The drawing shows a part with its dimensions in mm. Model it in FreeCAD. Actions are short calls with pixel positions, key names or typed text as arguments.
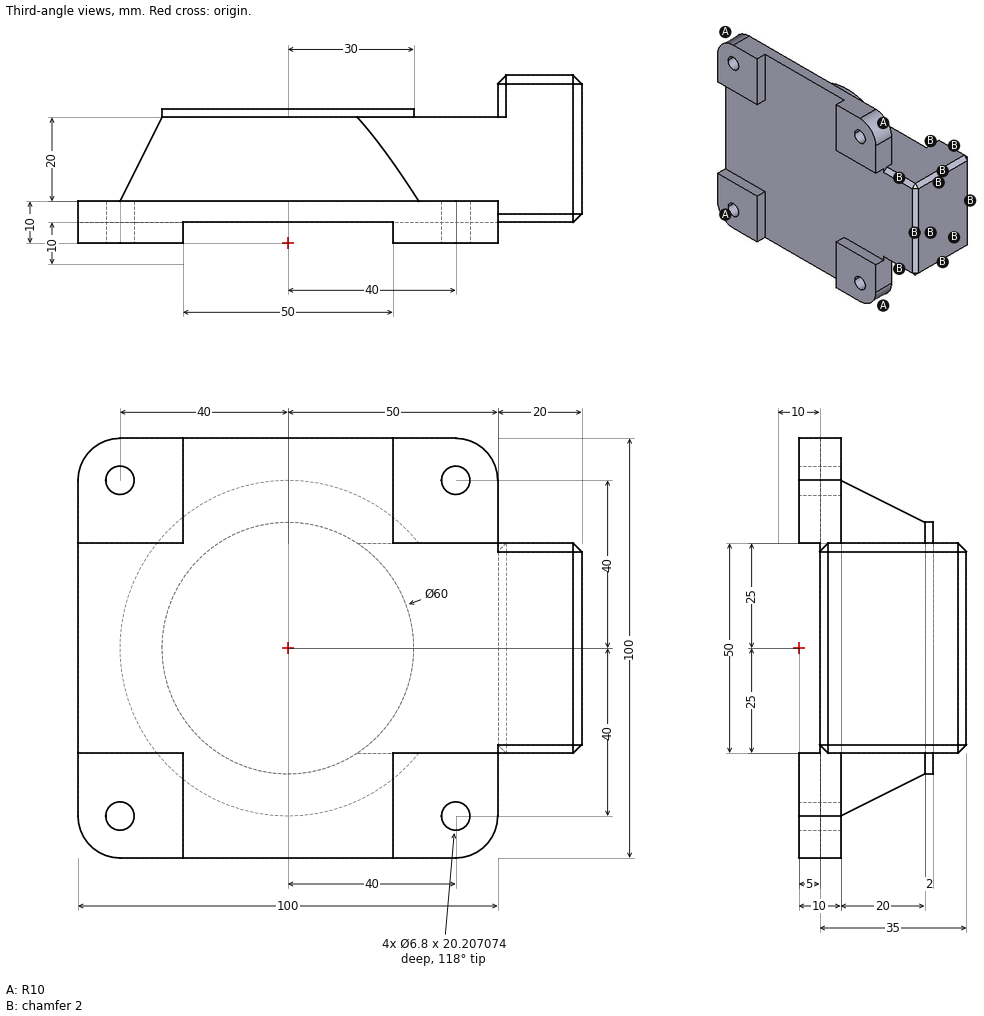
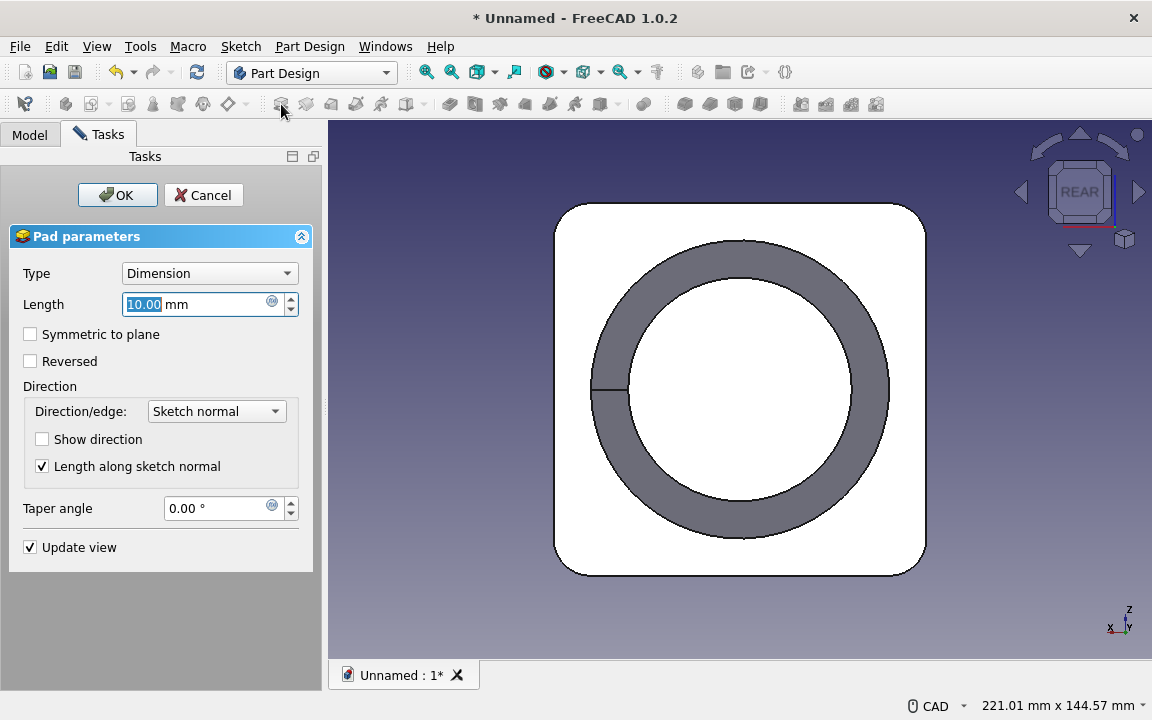
text(2)
key(Tab)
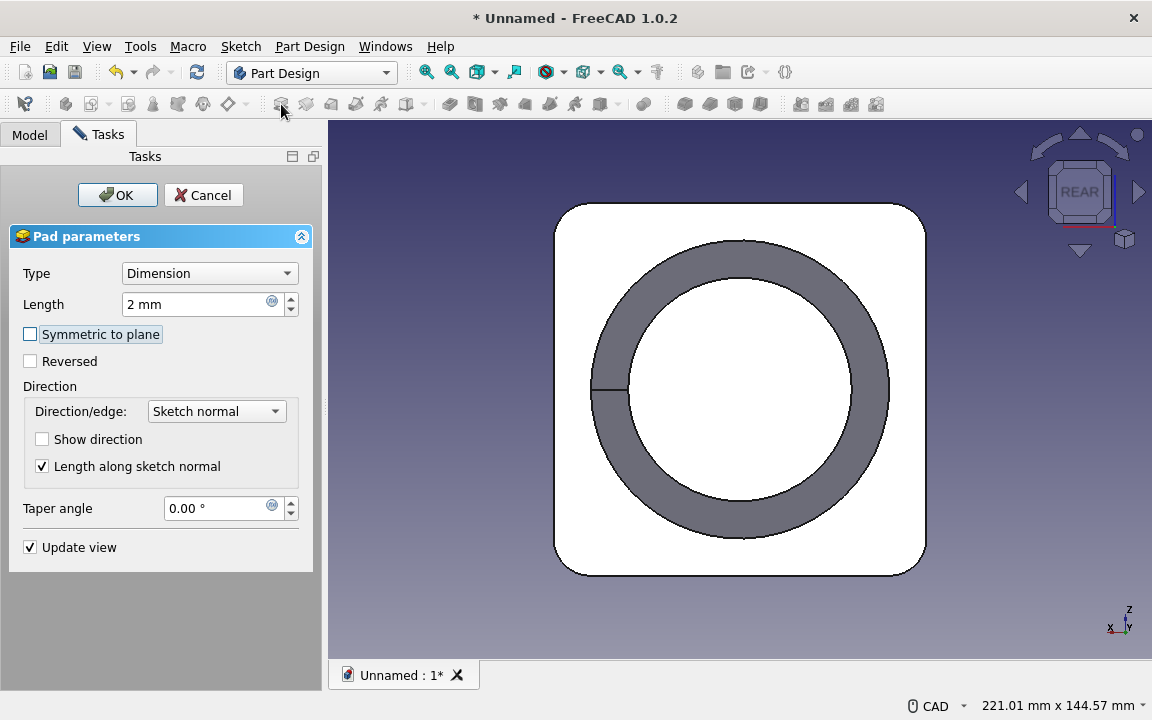
click(118, 195)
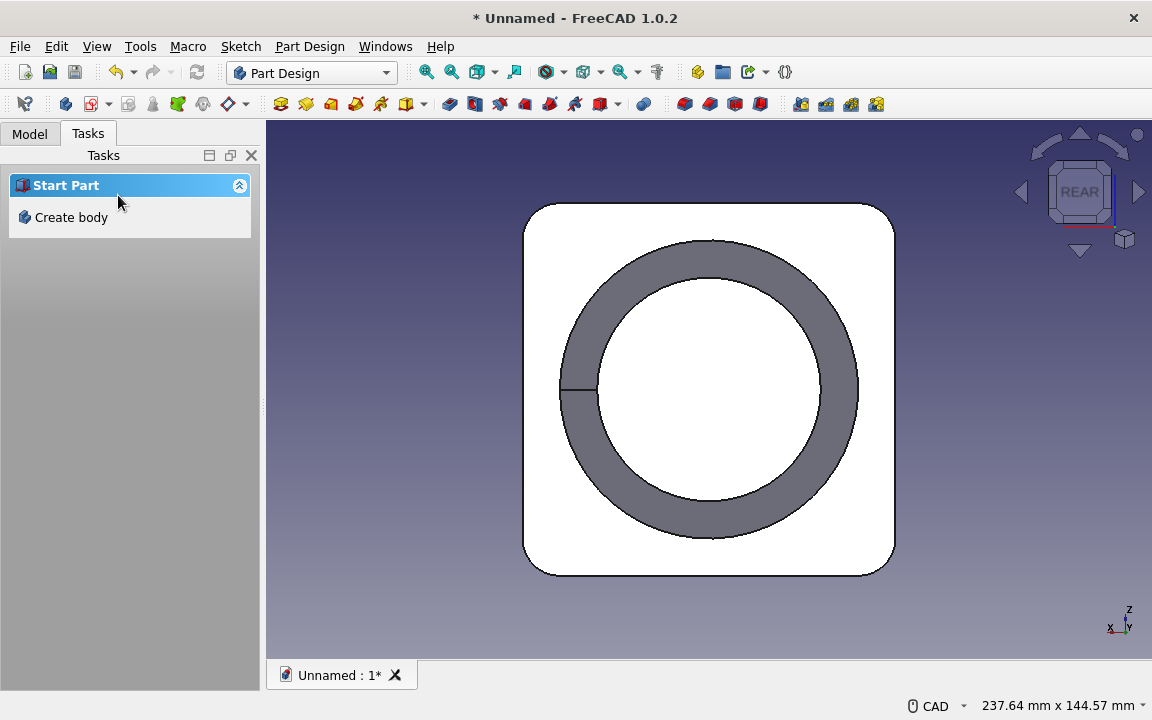
click(90, 104)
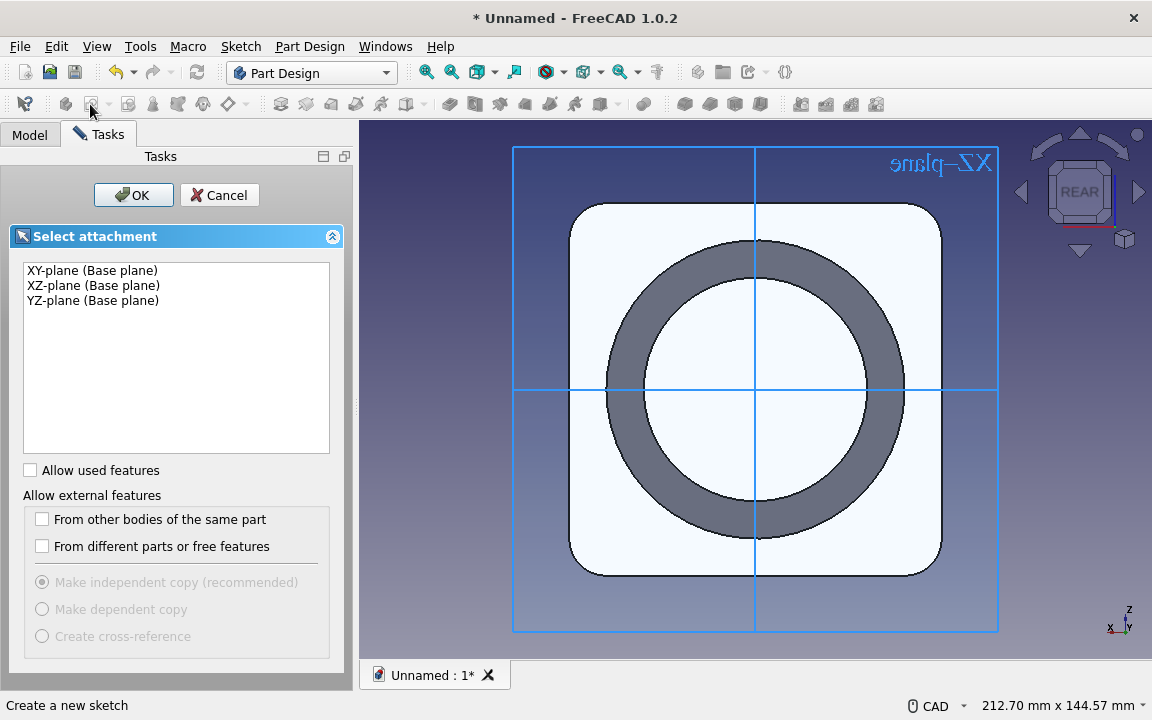
click(84, 300)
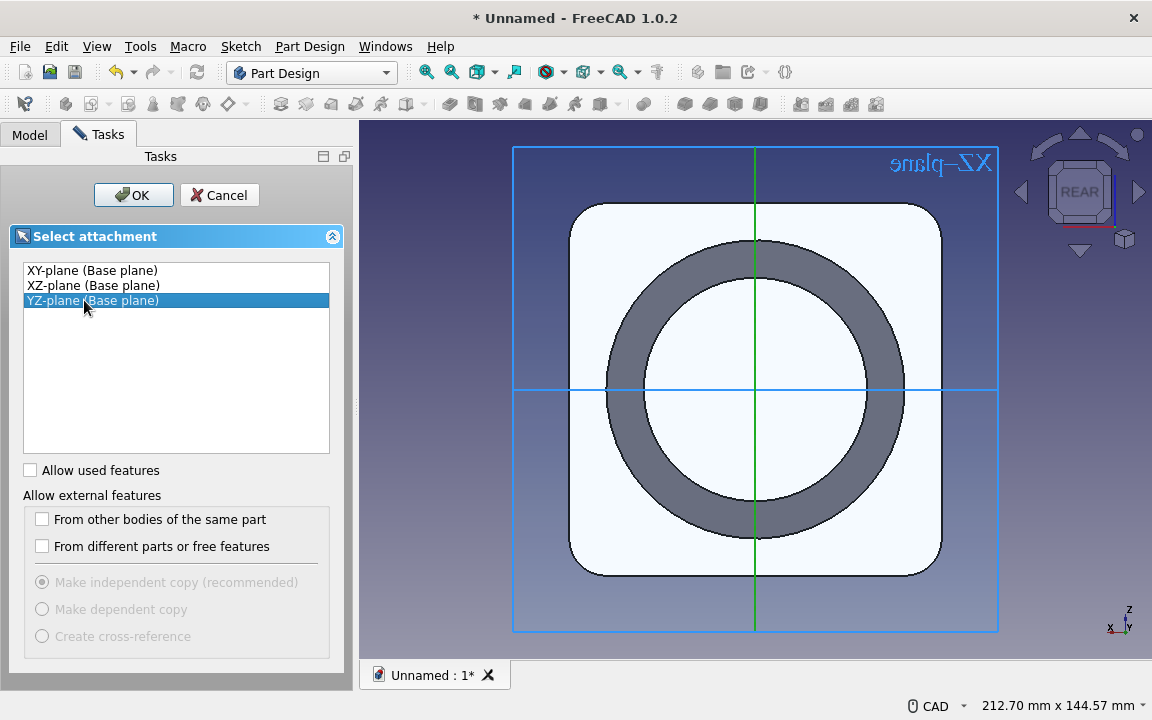
click(134, 195)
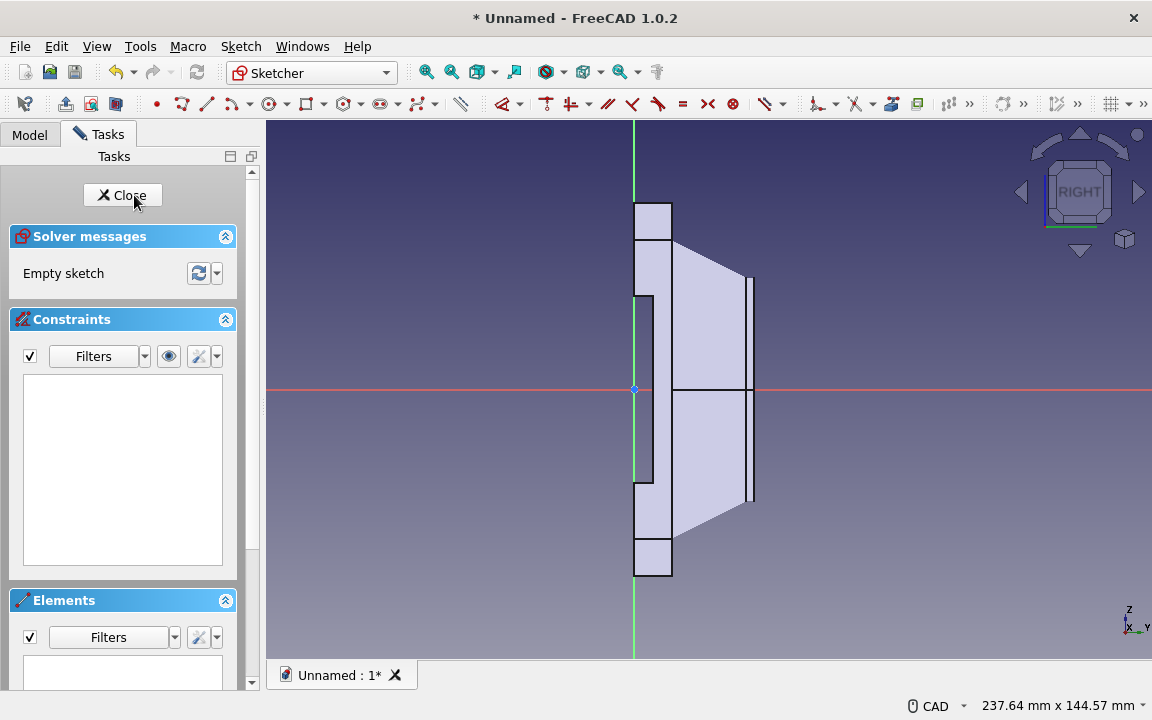
key(q)
key(s)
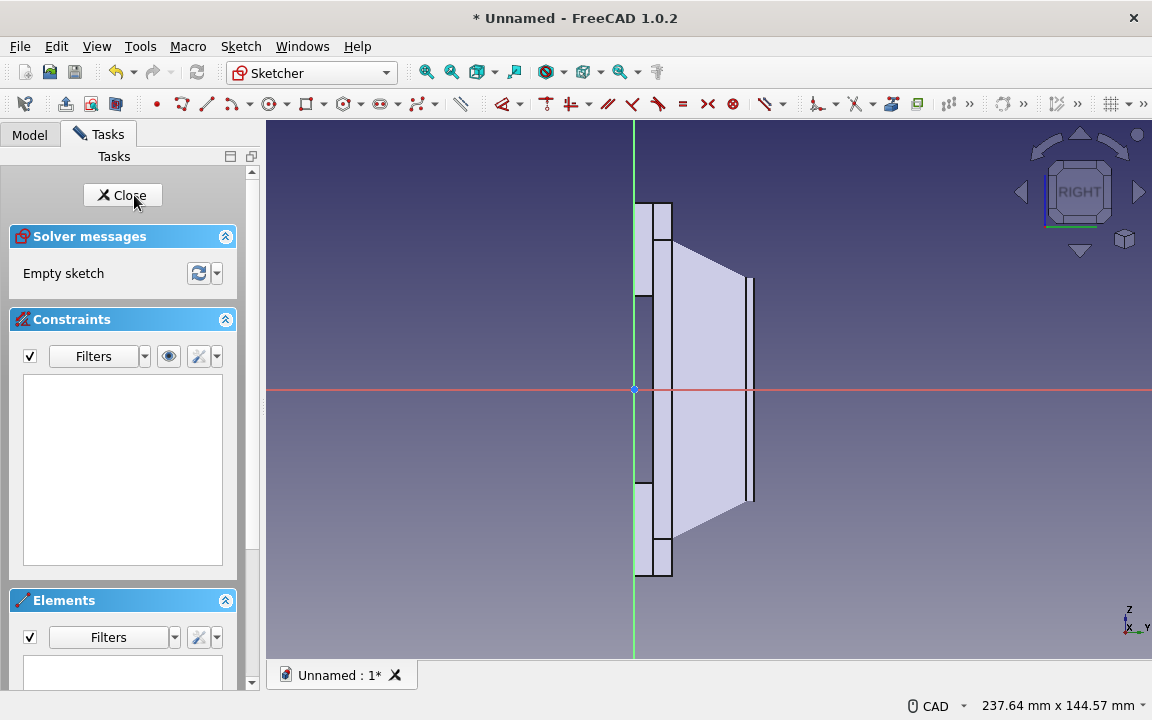
scroll(751, 390, up, 3)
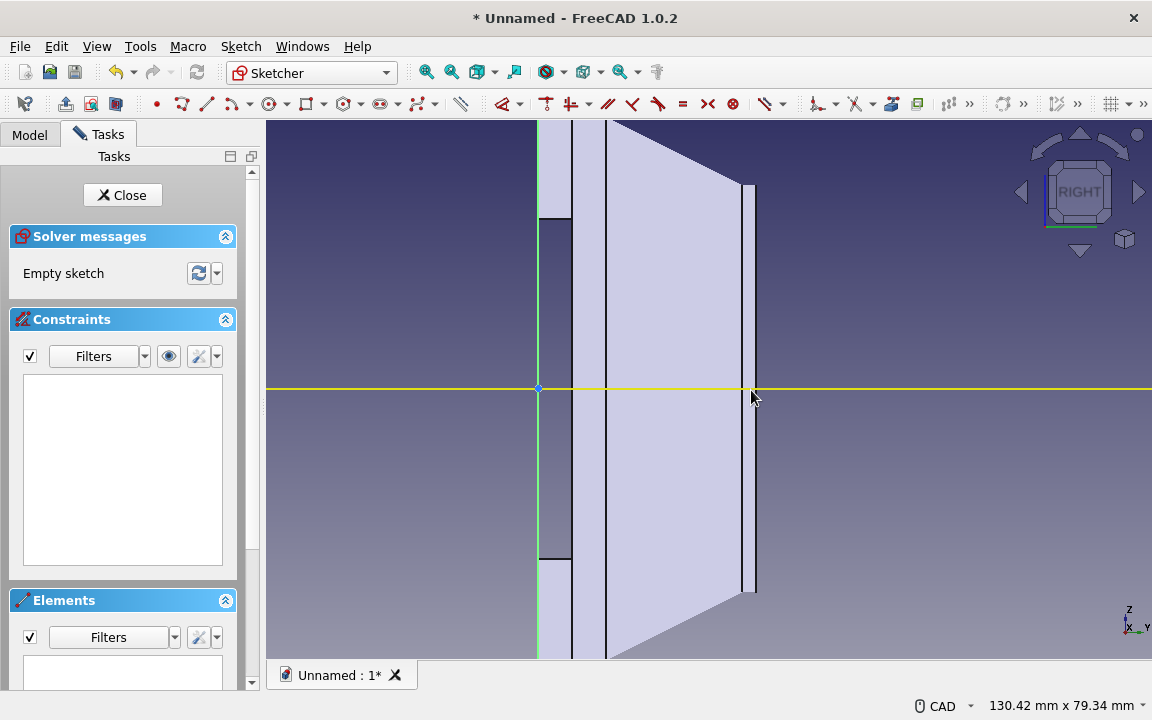
click(306, 104)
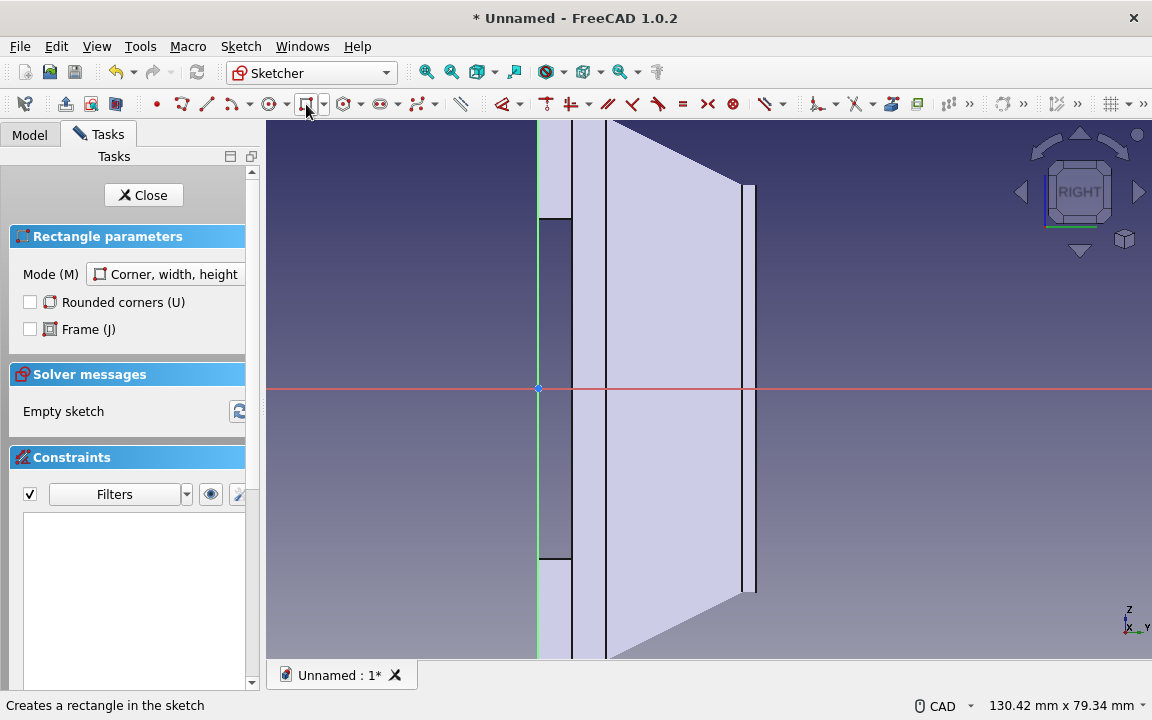
click(606, 219)
click(742, 559)
key(Escape)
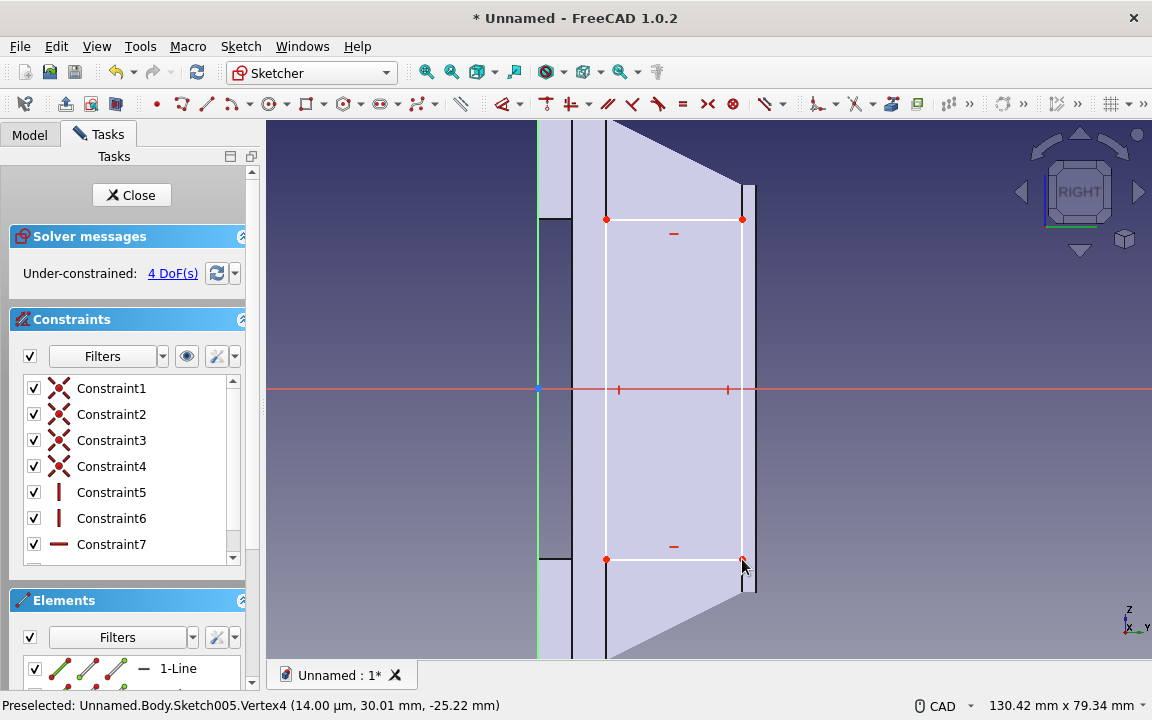
click(502, 104)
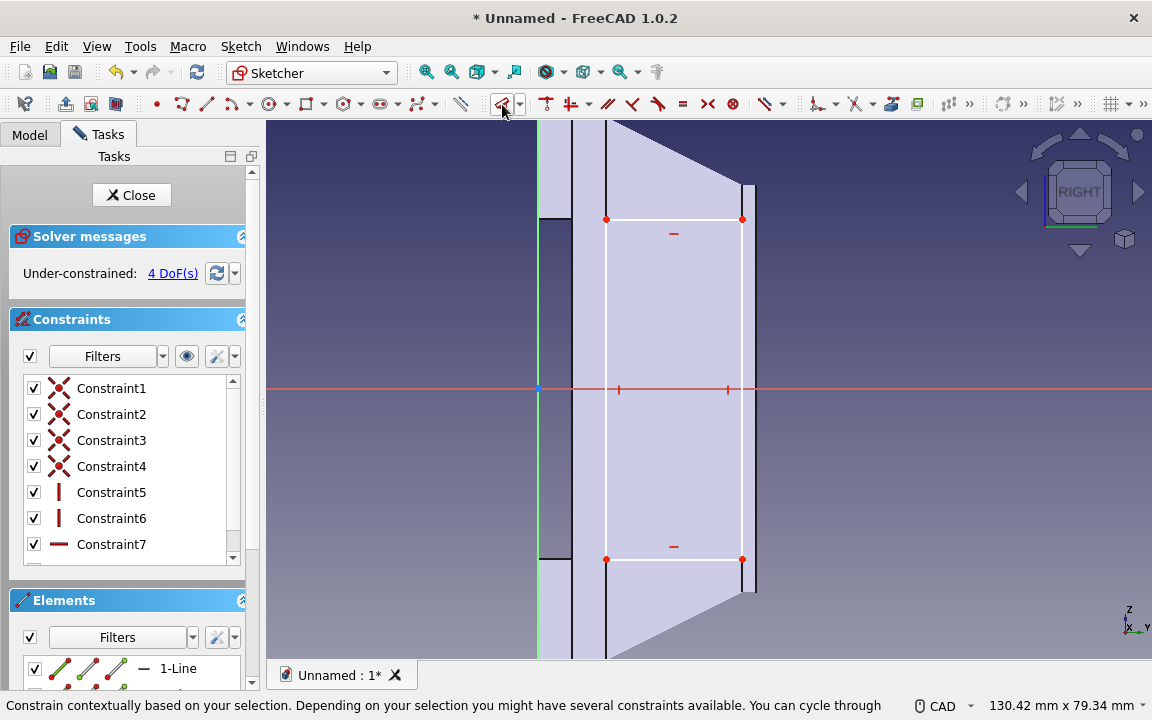
click(606, 322)
click(572, 312)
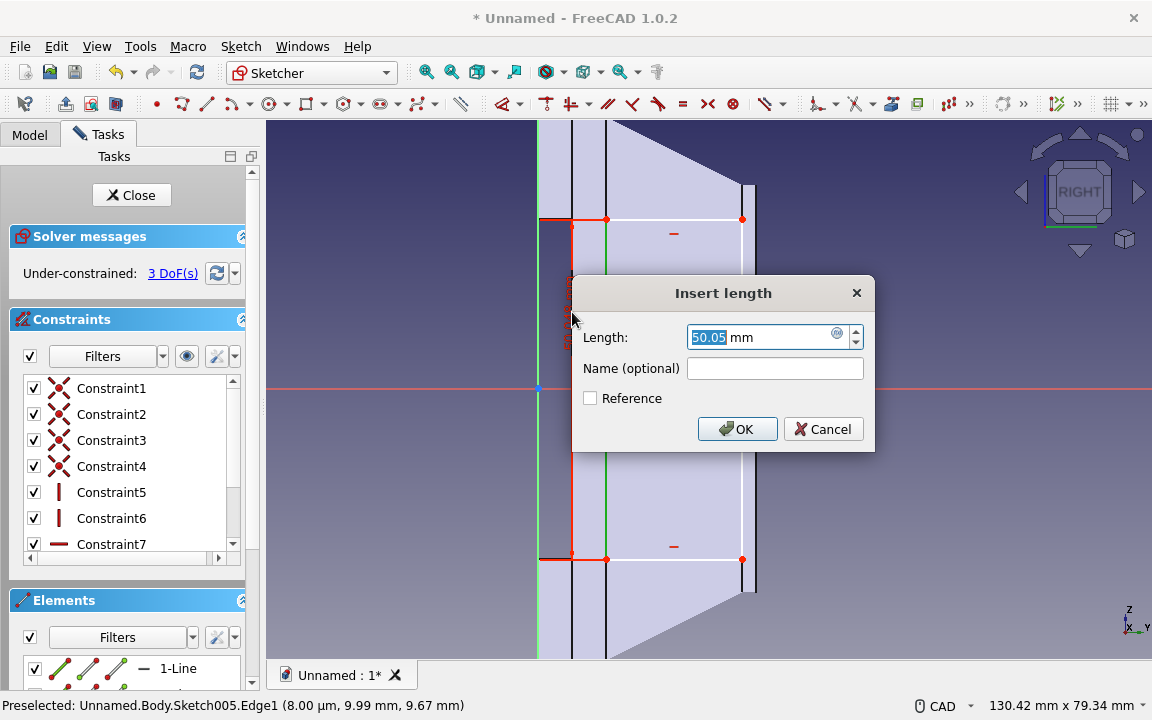
text(50)
key(Return)